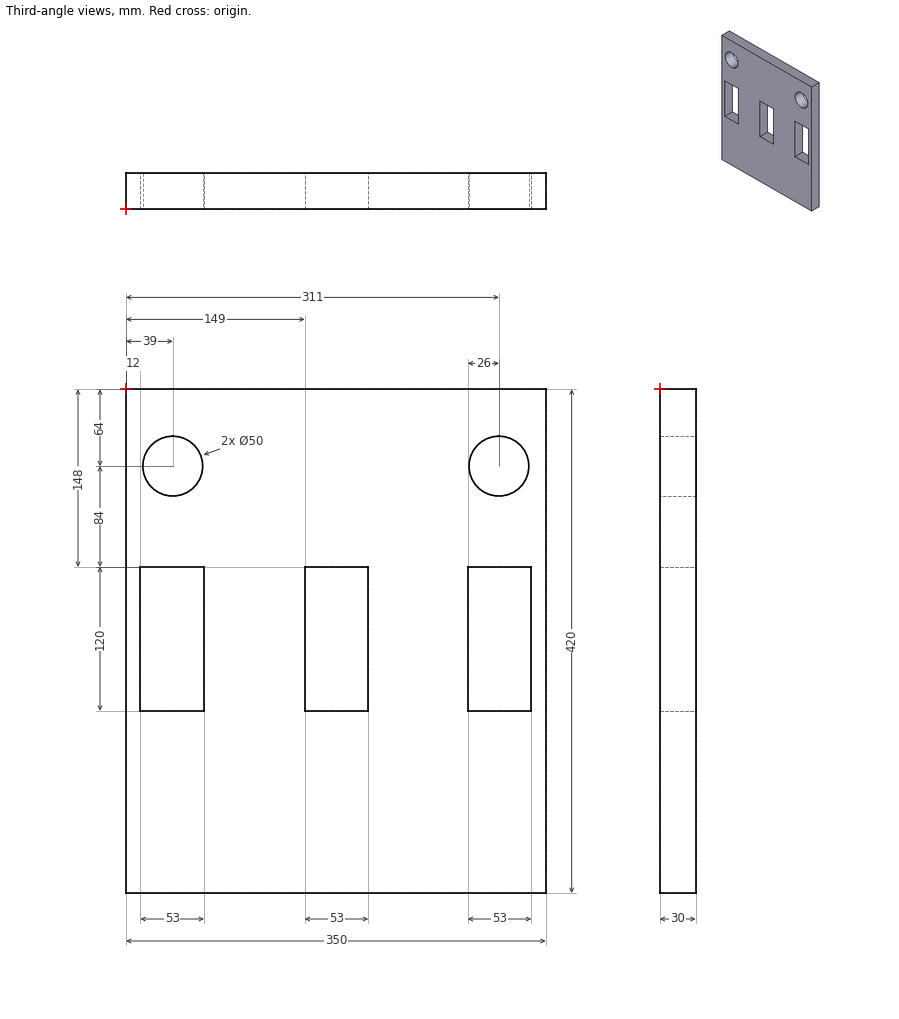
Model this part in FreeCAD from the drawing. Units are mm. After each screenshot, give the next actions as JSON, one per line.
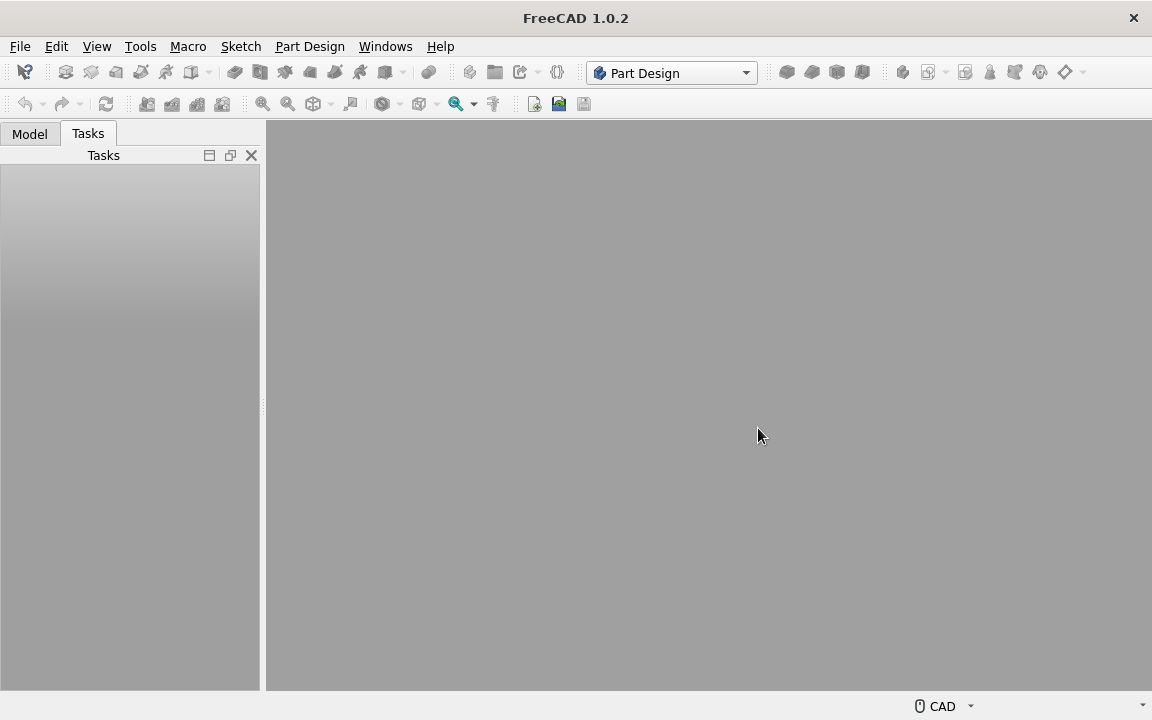
{"action": "left_click", "coordinate": [534, 104]}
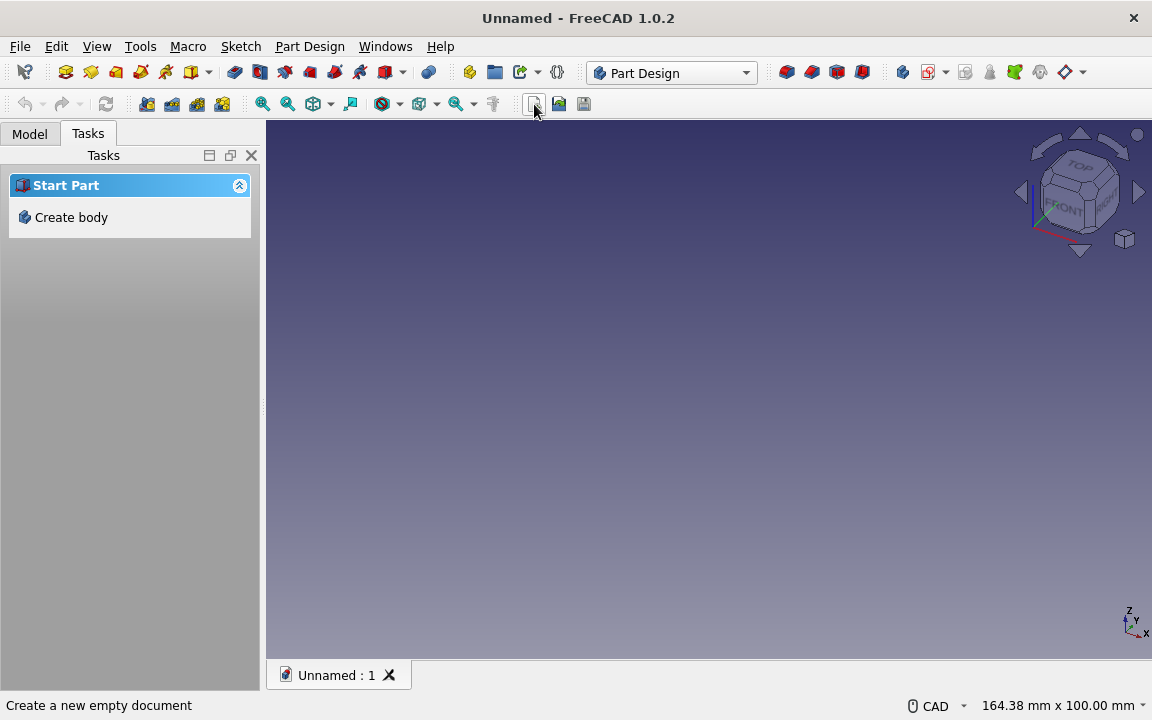
{"action": "left_click", "coordinate": [928, 72]}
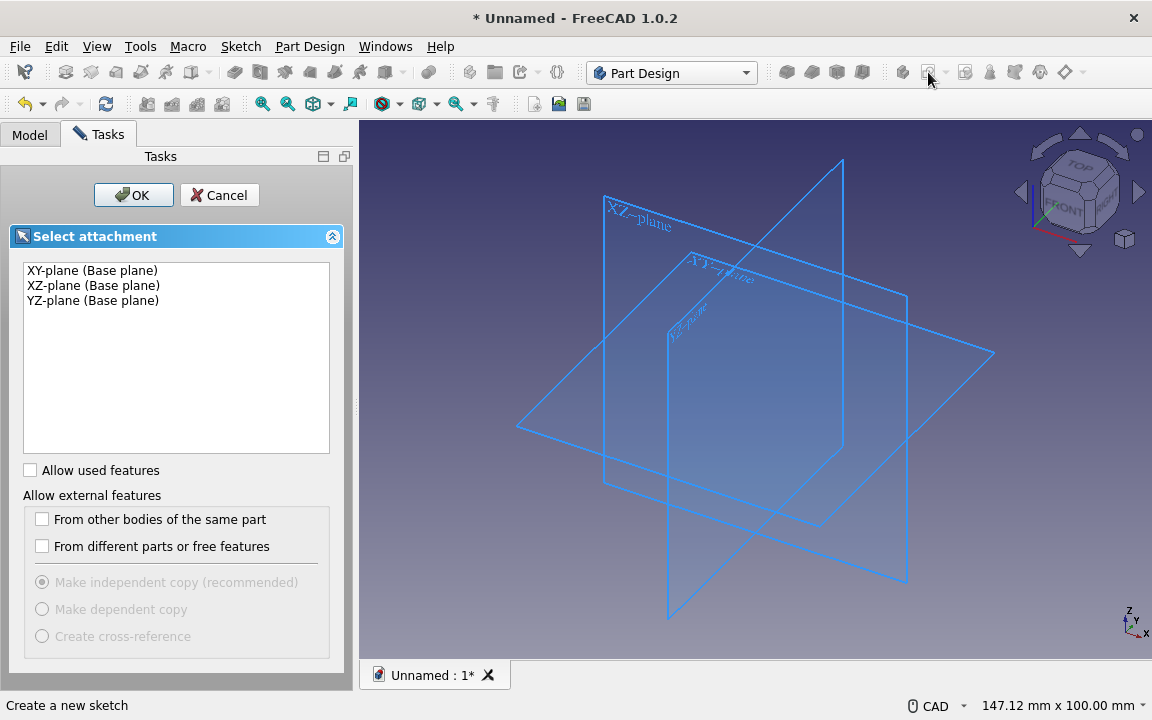
{"action": "left_click", "coordinate": [84, 286]}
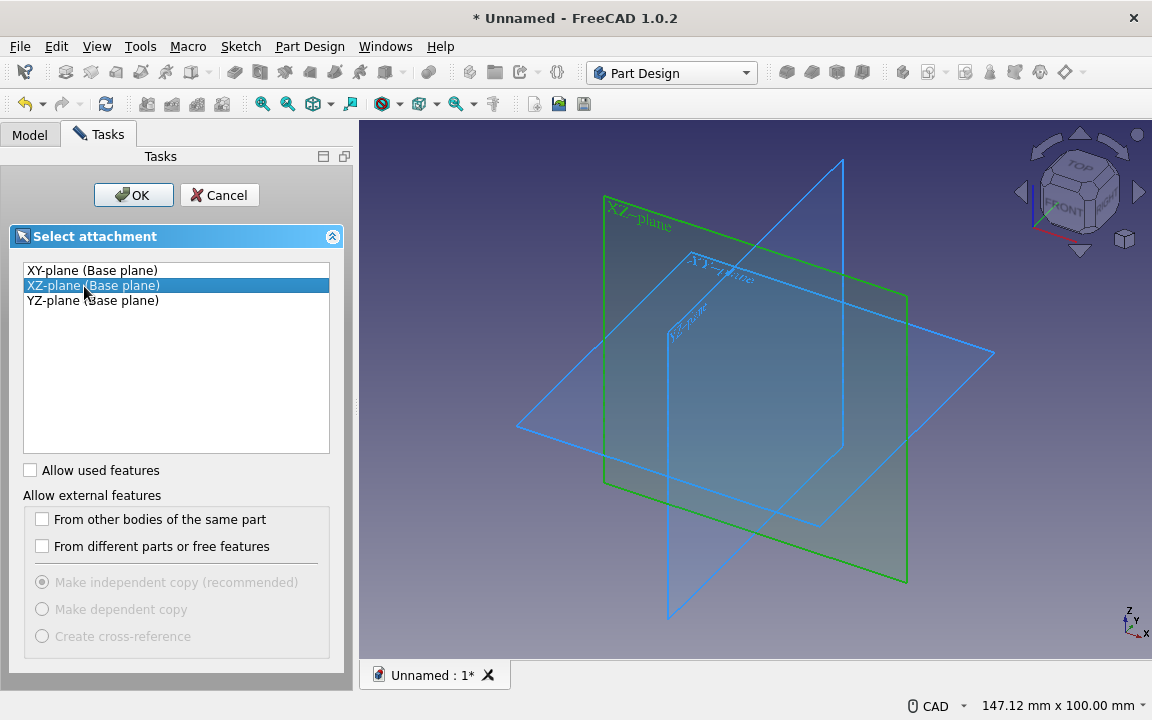
{"action": "left_click", "coordinate": [134, 195]}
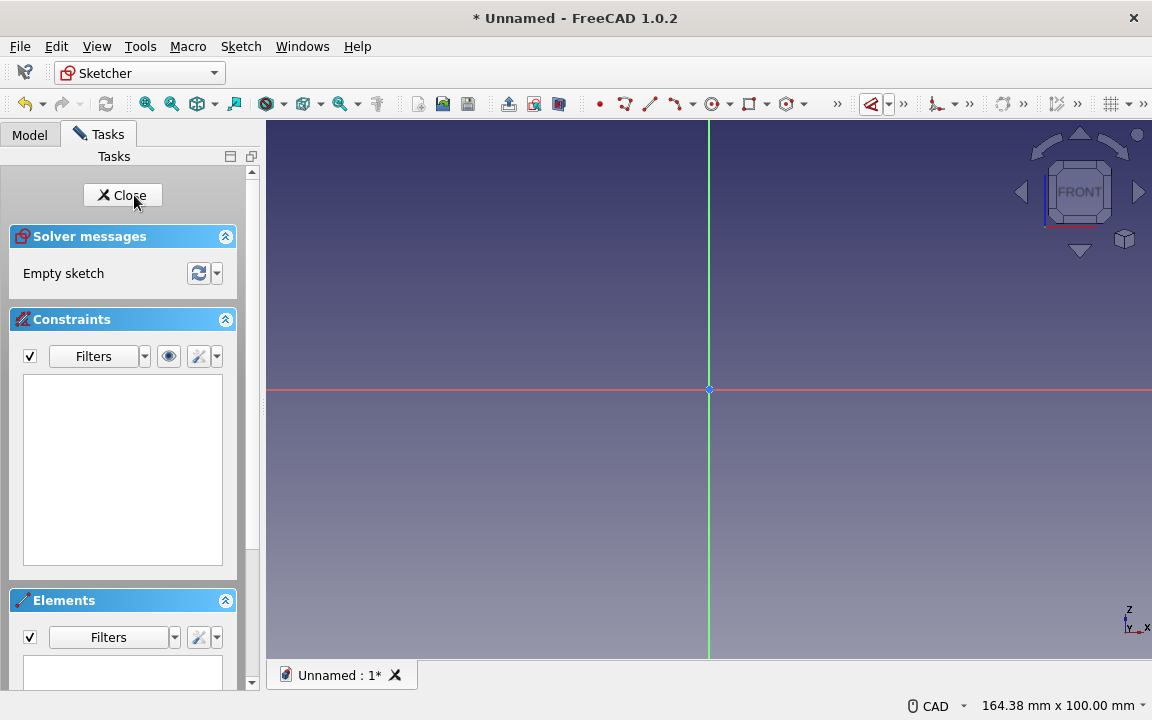
{"action": "scroll", "coordinate": [440, 165], "scroll_direction": "down", "scroll_amount": 9}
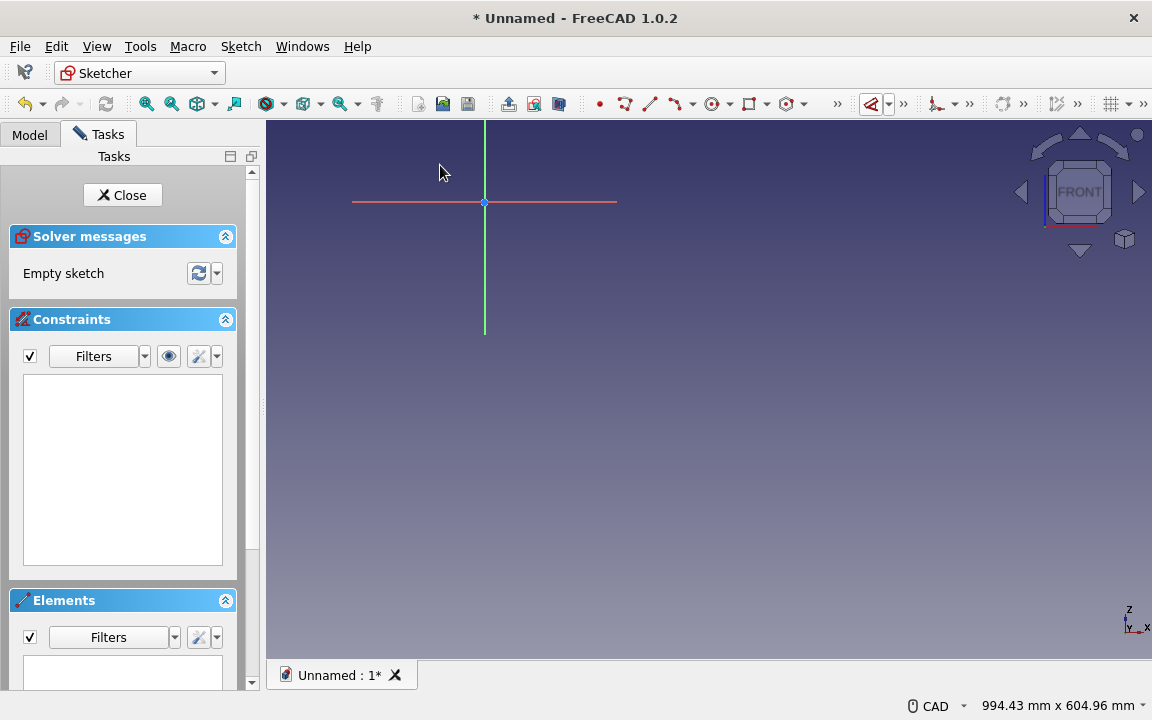
{"action": "left_click", "coordinate": [748, 104]}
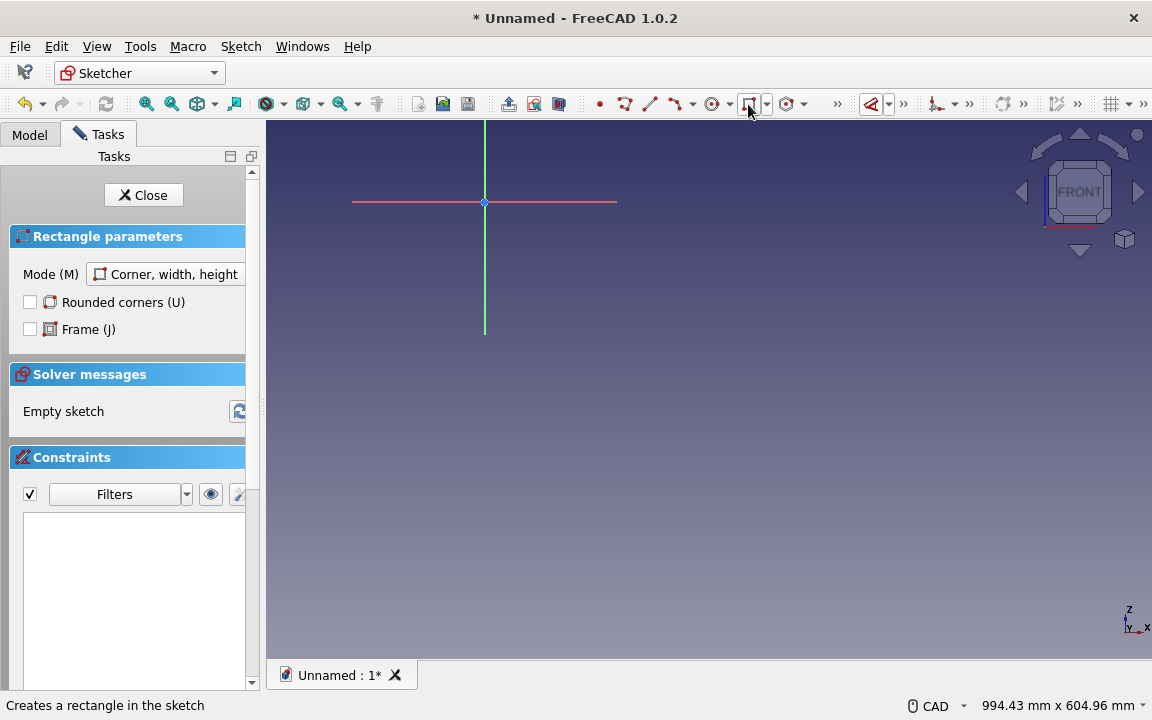
{"action": "left_click", "coordinate": [485, 202]}
{"action": "mouse_move", "coordinate": [796, 576]}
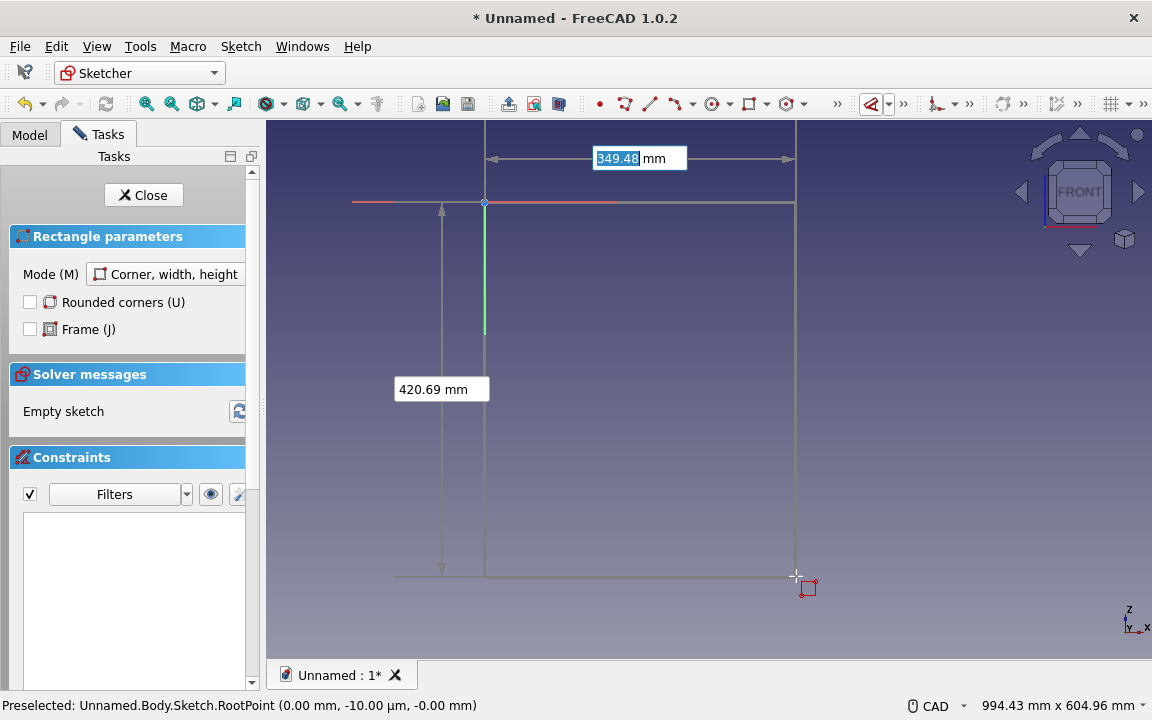
{"action": "type", "text": "350"}
{"action": "key", "text": "Tab"}
{"action": "type", "text": "420"}
{"action": "key", "text": "Return"}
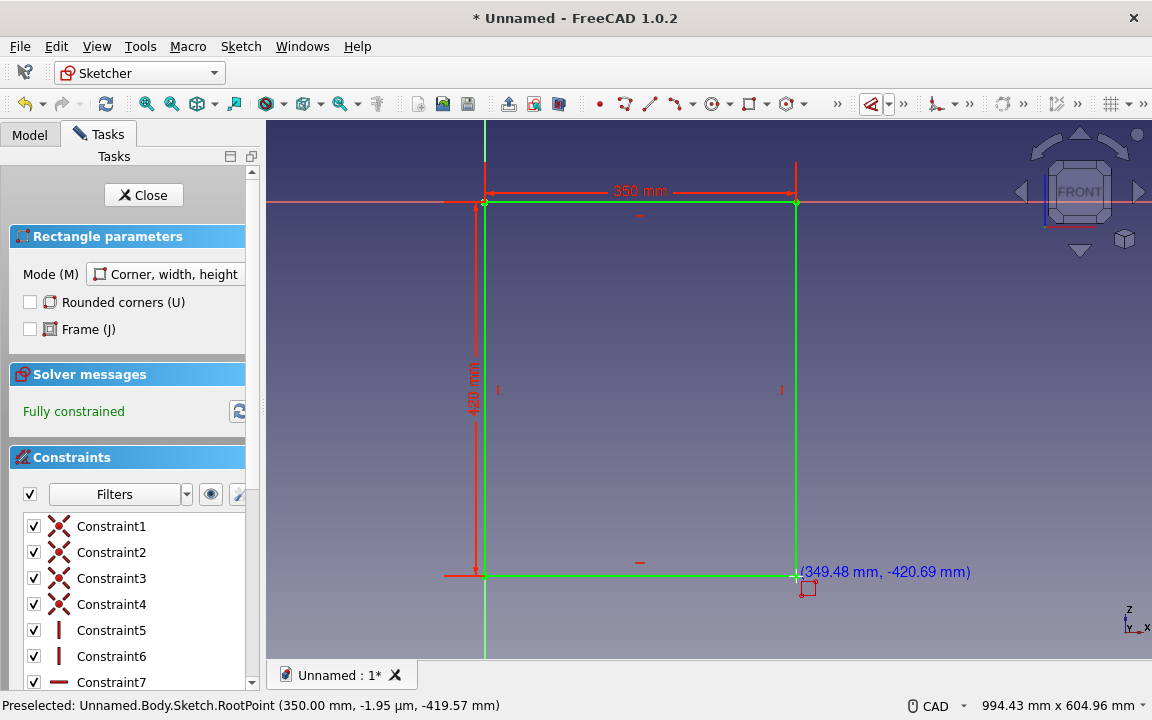
{"action": "scroll", "coordinate": [495, 334], "scroll_direction": "up", "scroll_amount": 2}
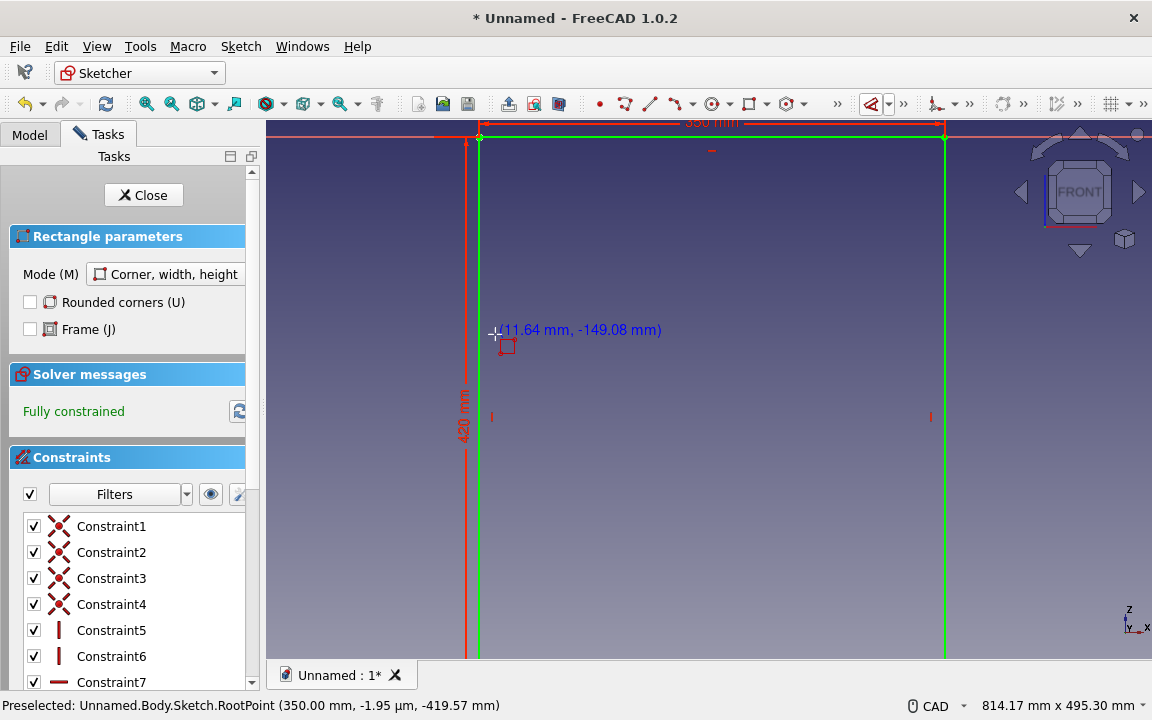
{"action": "left_click", "coordinate": [495, 334]}
{"action": "mouse_move", "coordinate": [566, 493]}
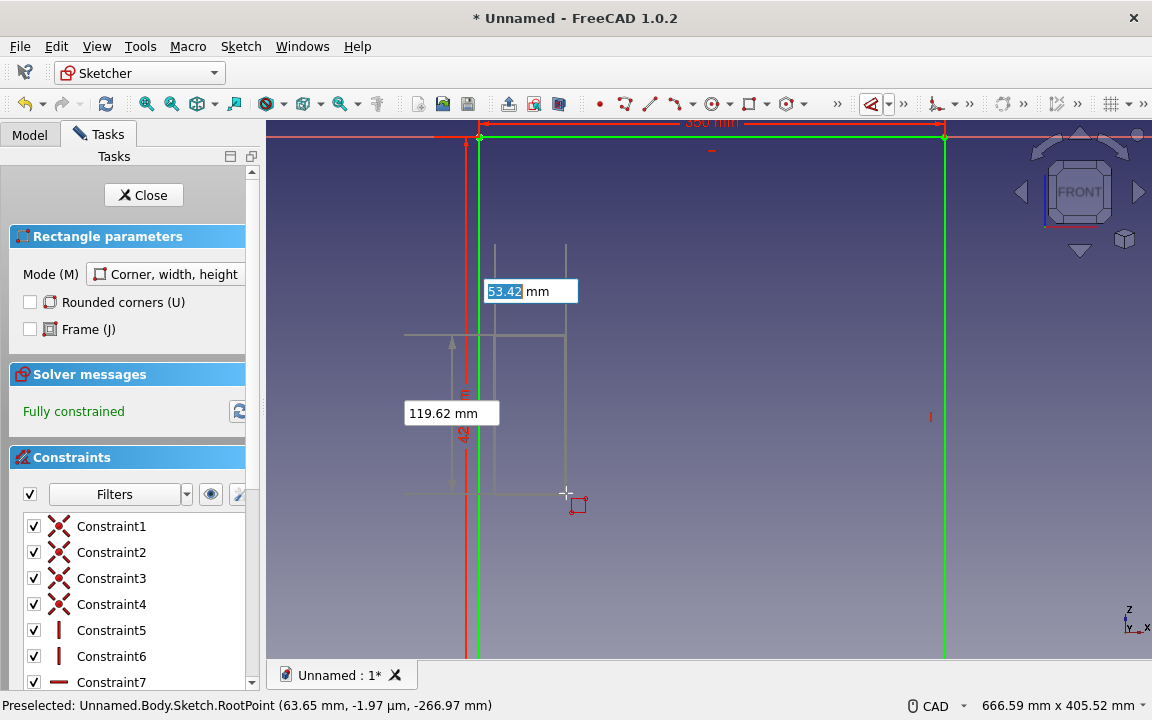
{"action": "type", "text": "53"}
{"action": "key", "text": "Tab"}
{"action": "type", "text": "120"}
{"action": "key", "text": "Return"}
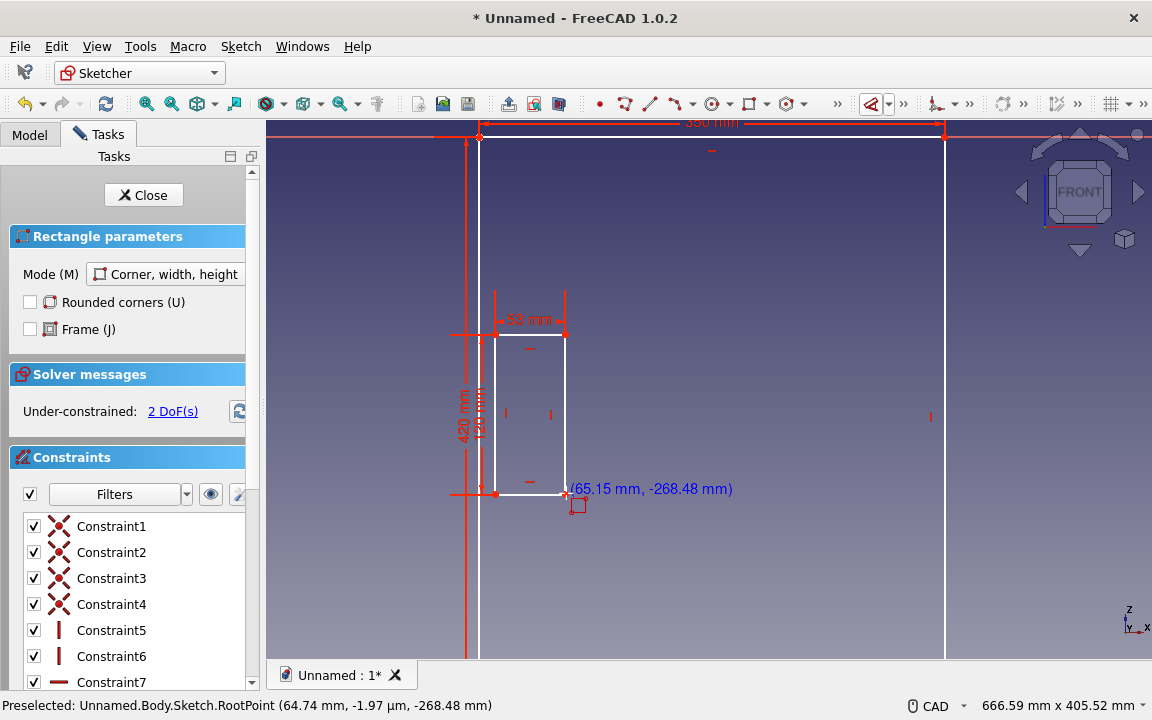
{"action": "left_click", "coordinate": [677, 334]}
{"action": "mouse_move", "coordinate": [748, 493]}